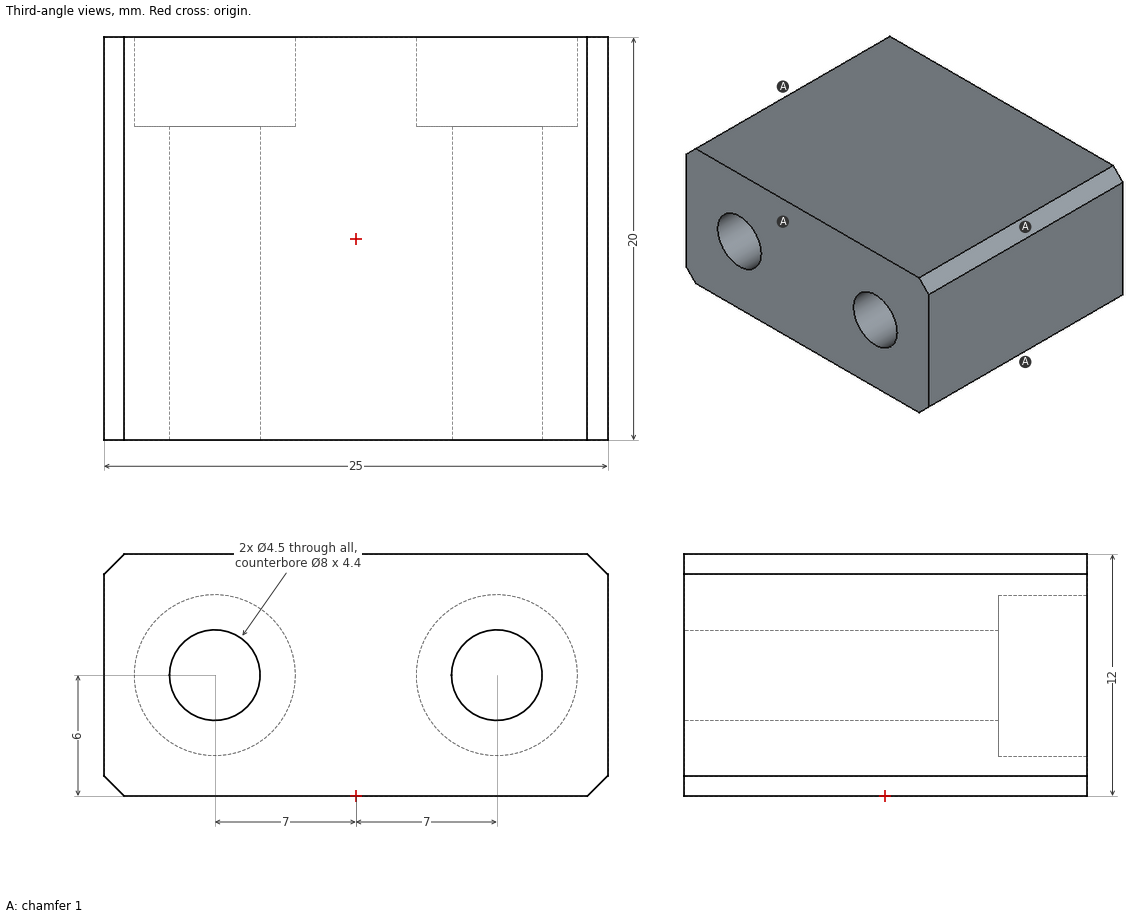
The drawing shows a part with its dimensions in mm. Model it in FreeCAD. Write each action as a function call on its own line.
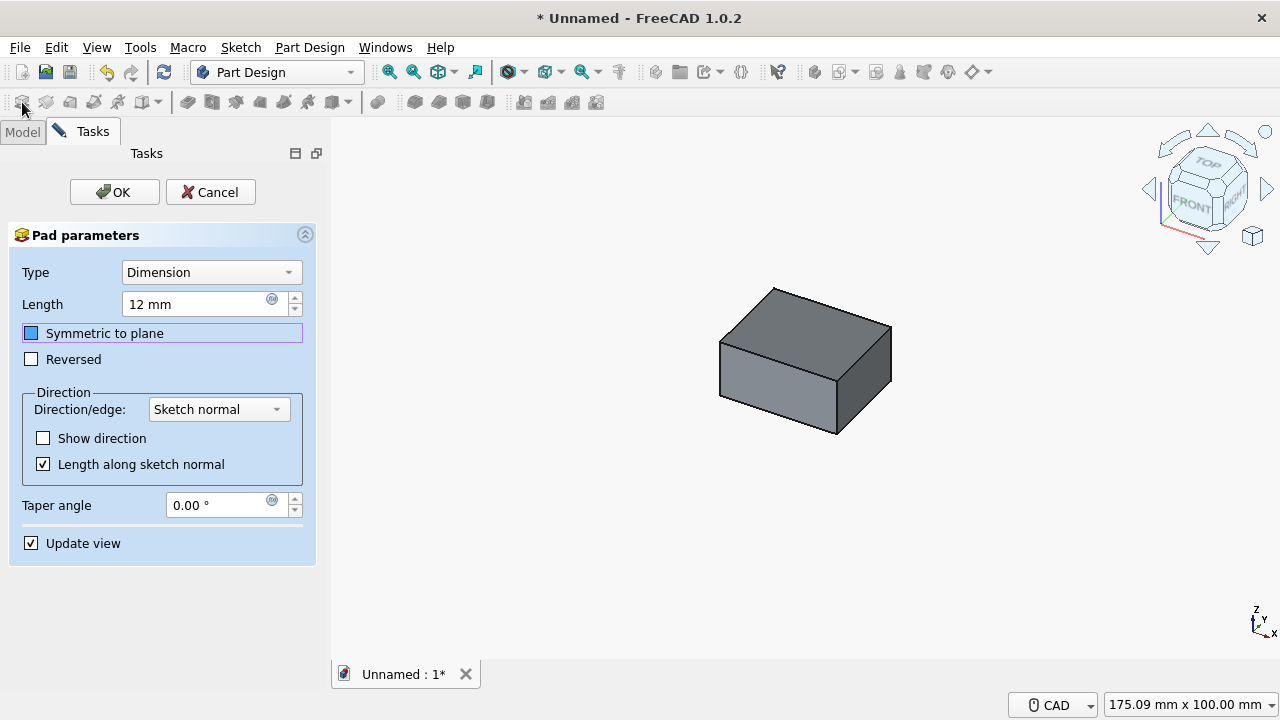
click(115, 192)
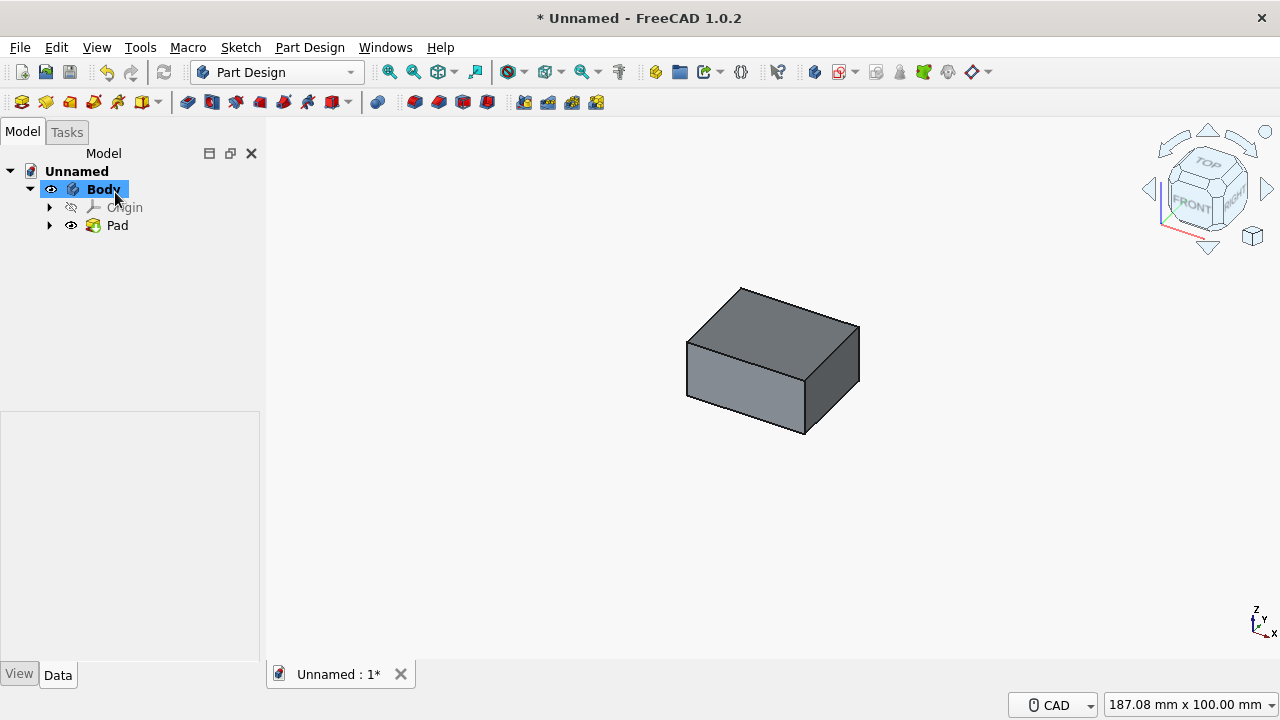
click(390, 72)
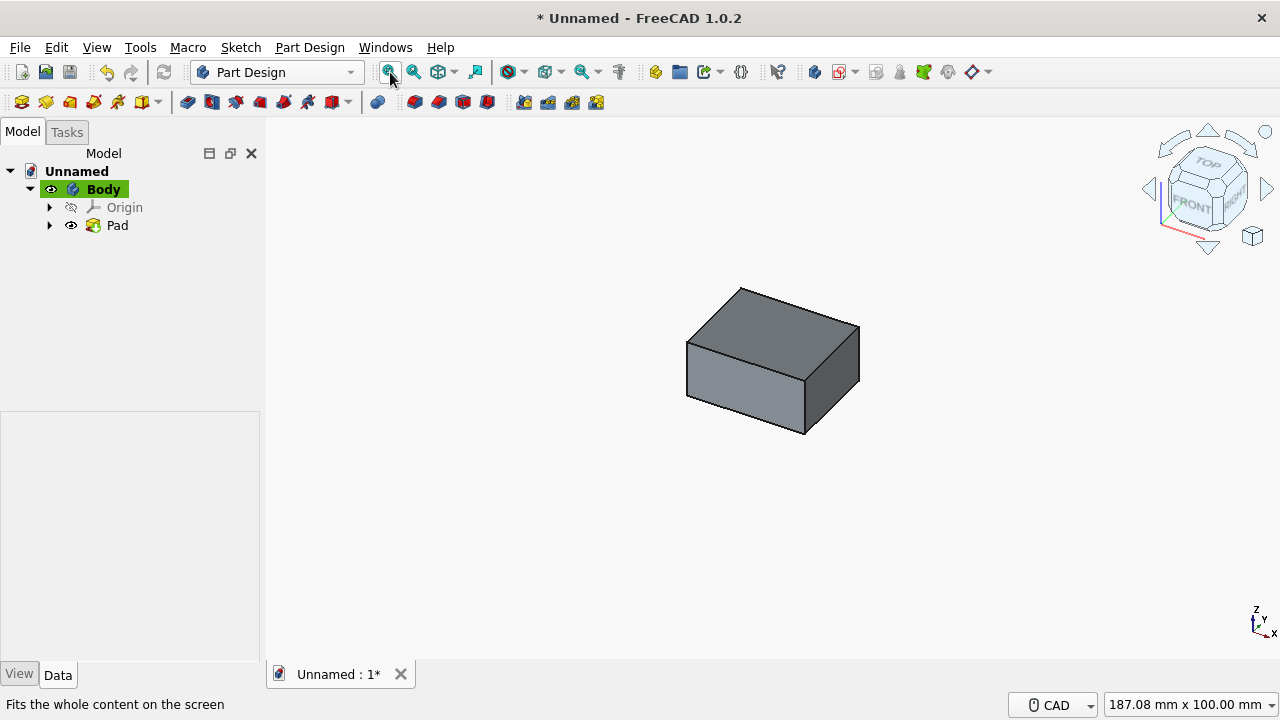
key(4)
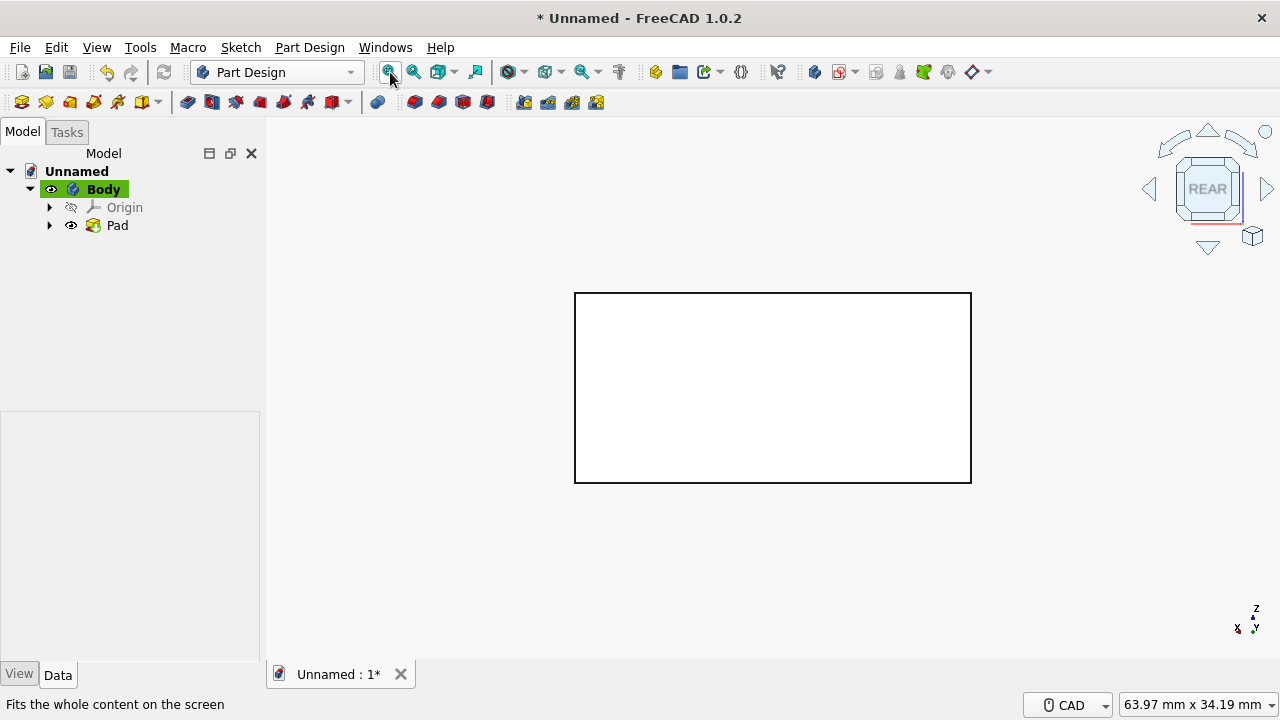
click(390, 72)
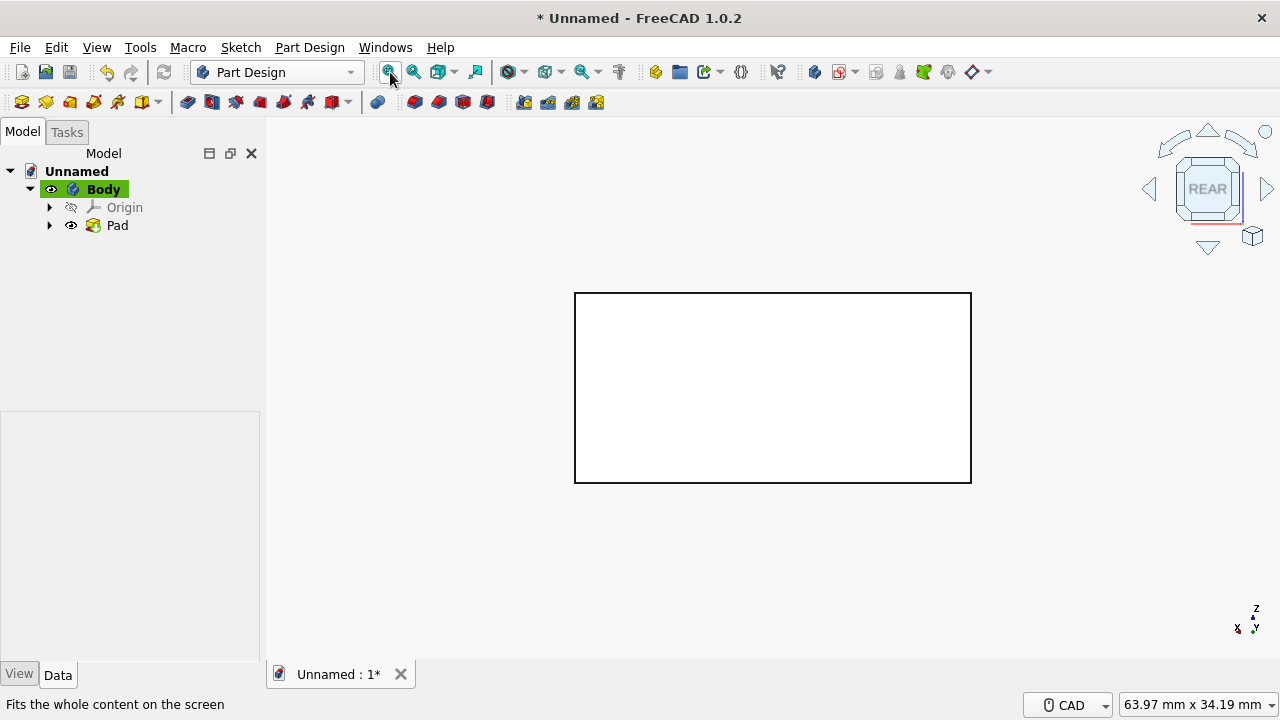
click(716, 387)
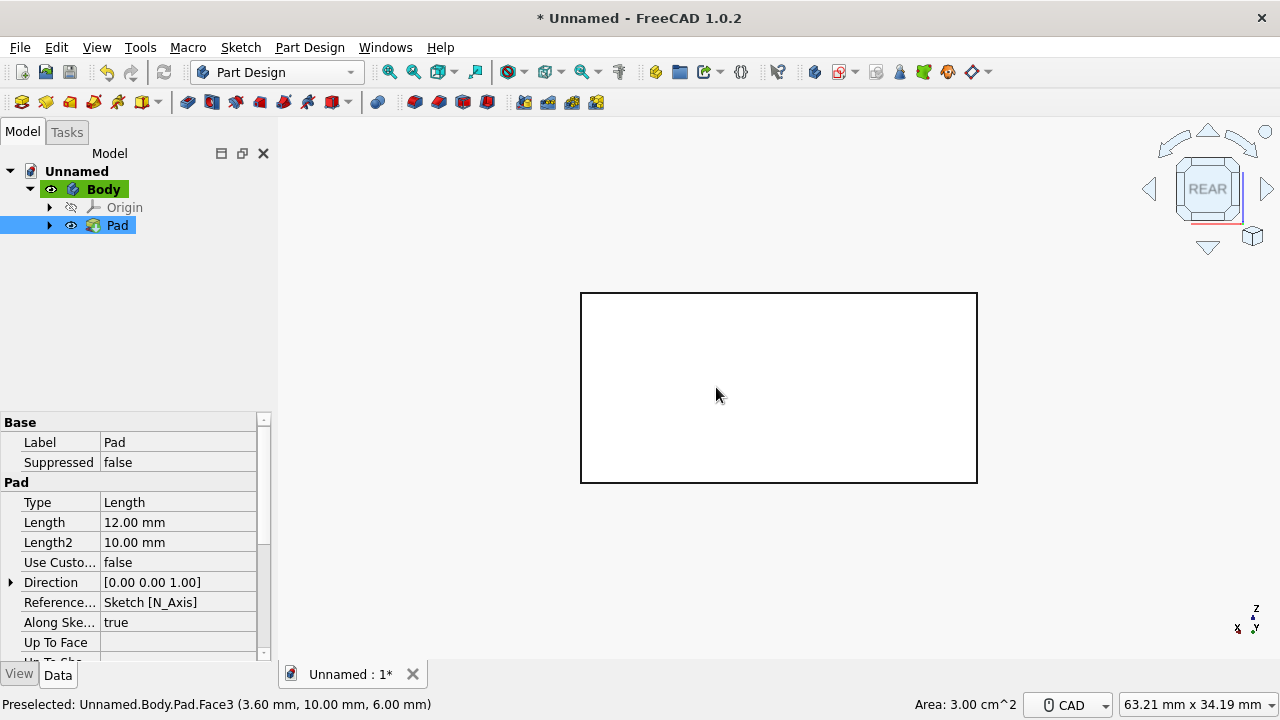
click(840, 72)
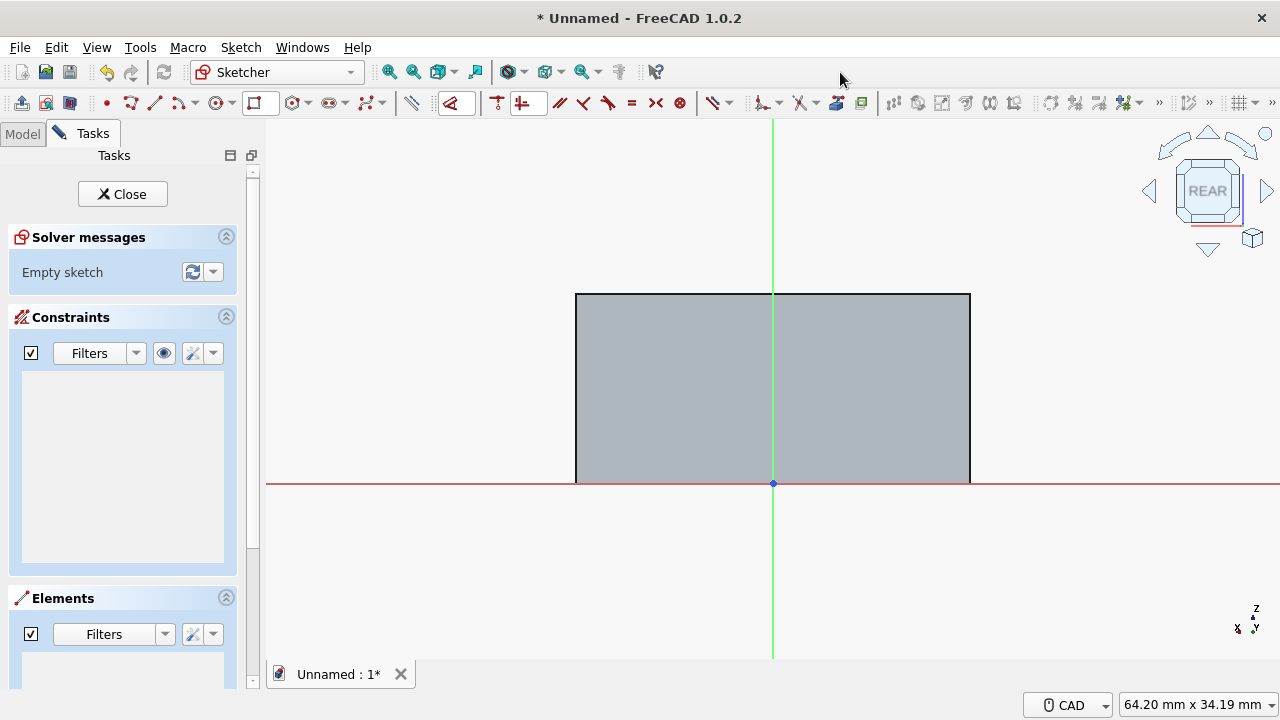
scroll(856, 455, up, 3)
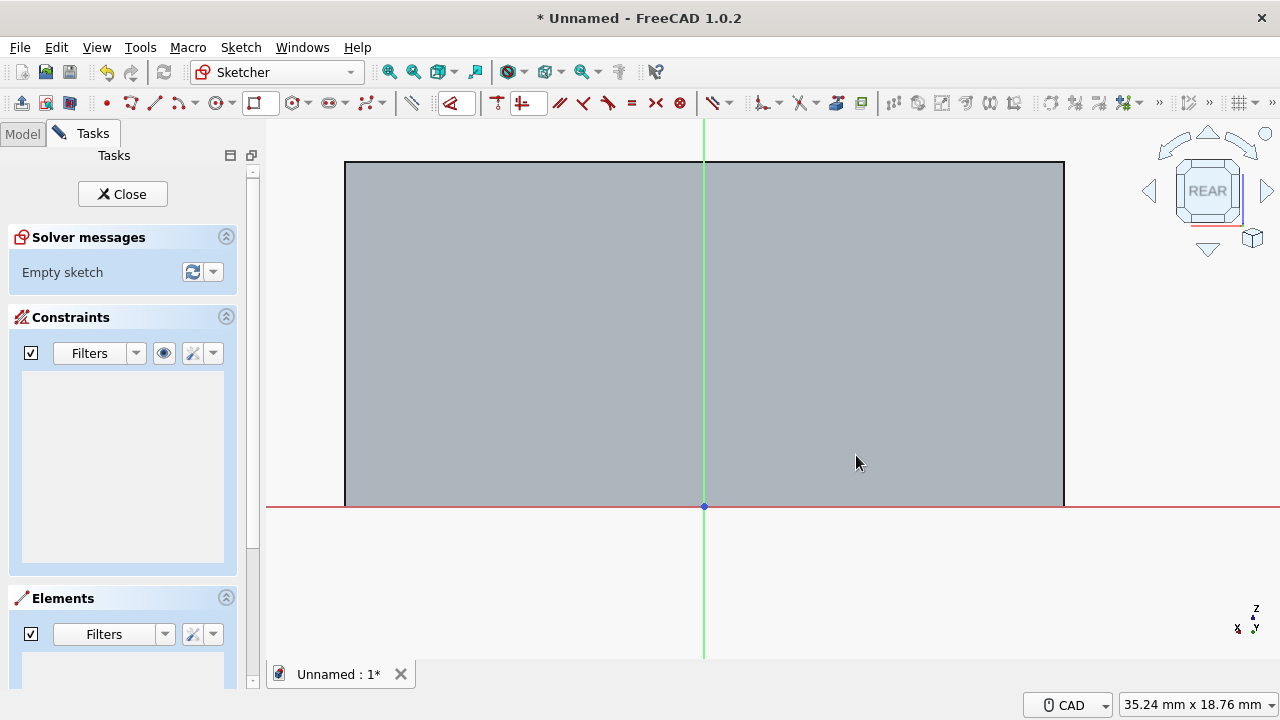
click(216, 104)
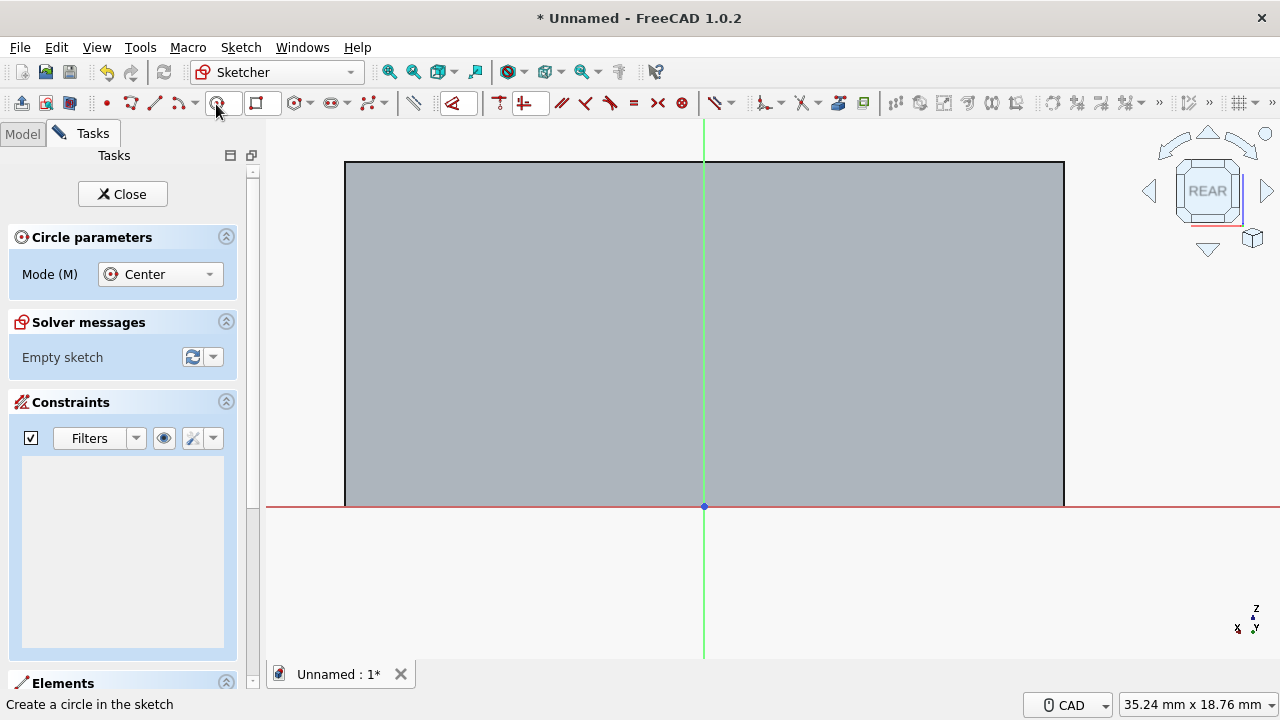
click(906, 334)
move(952, 288)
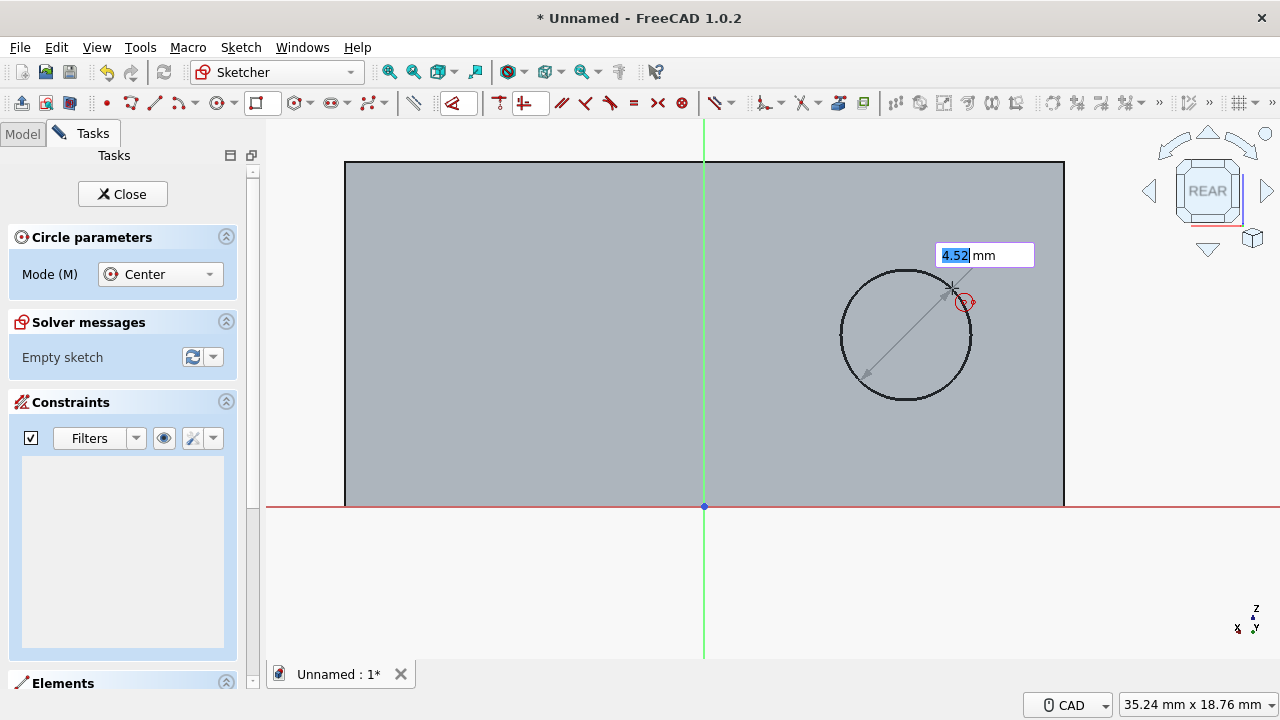
text(4.5)
key(Return)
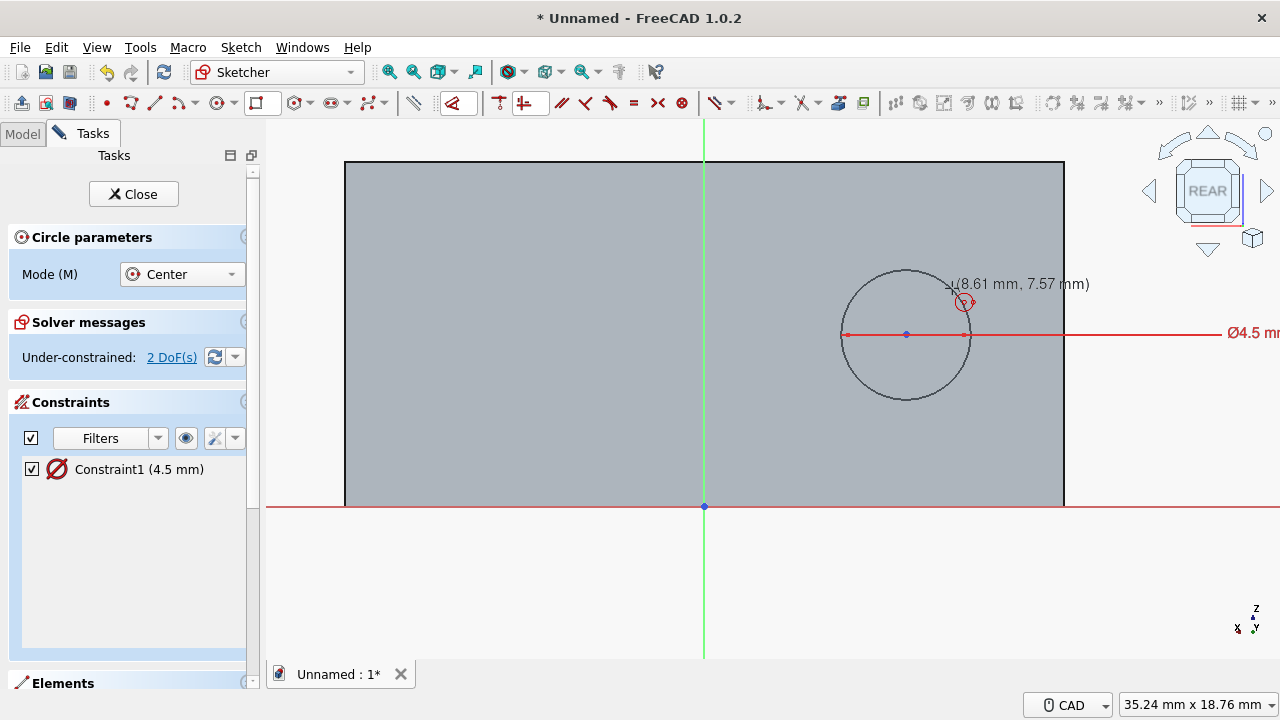
click(503, 334)
move(549, 288)